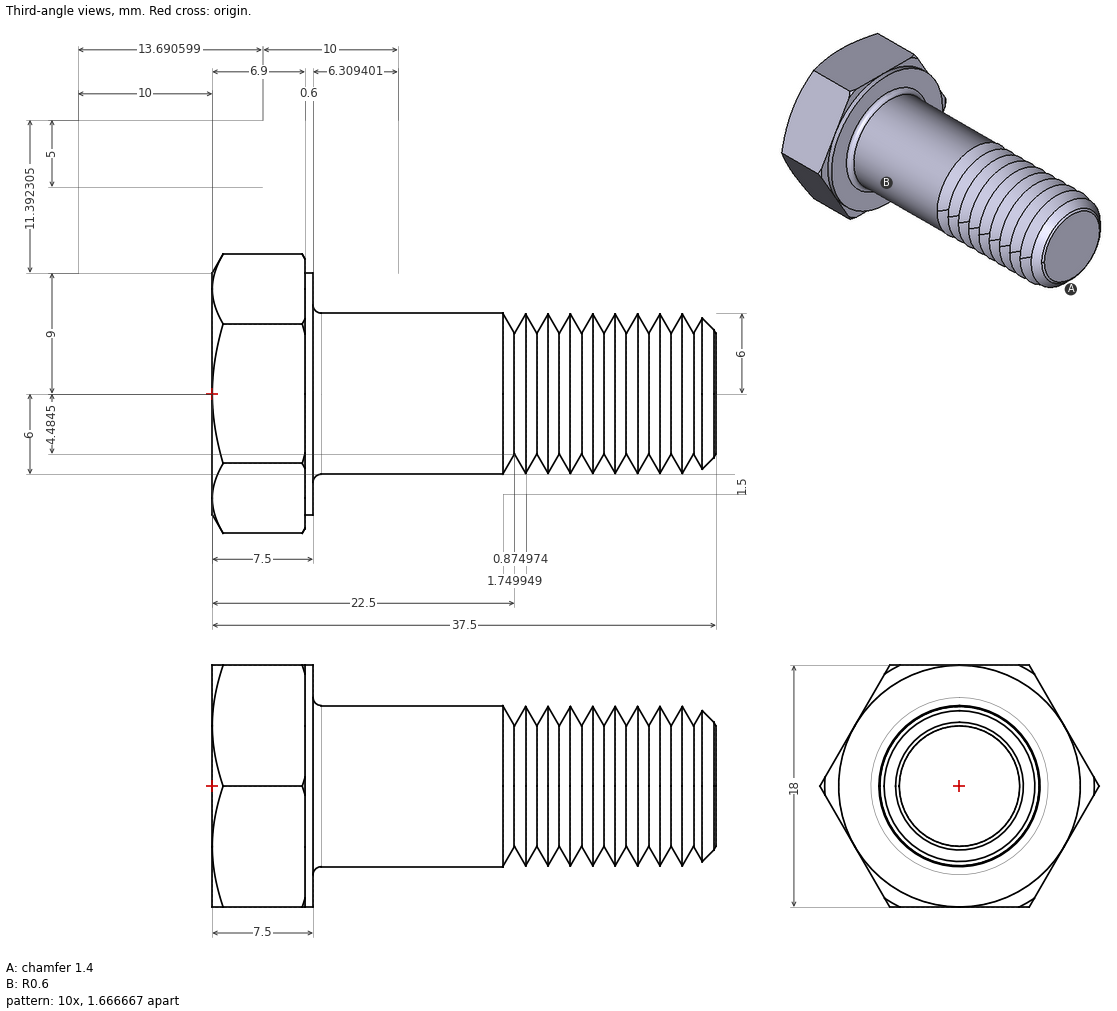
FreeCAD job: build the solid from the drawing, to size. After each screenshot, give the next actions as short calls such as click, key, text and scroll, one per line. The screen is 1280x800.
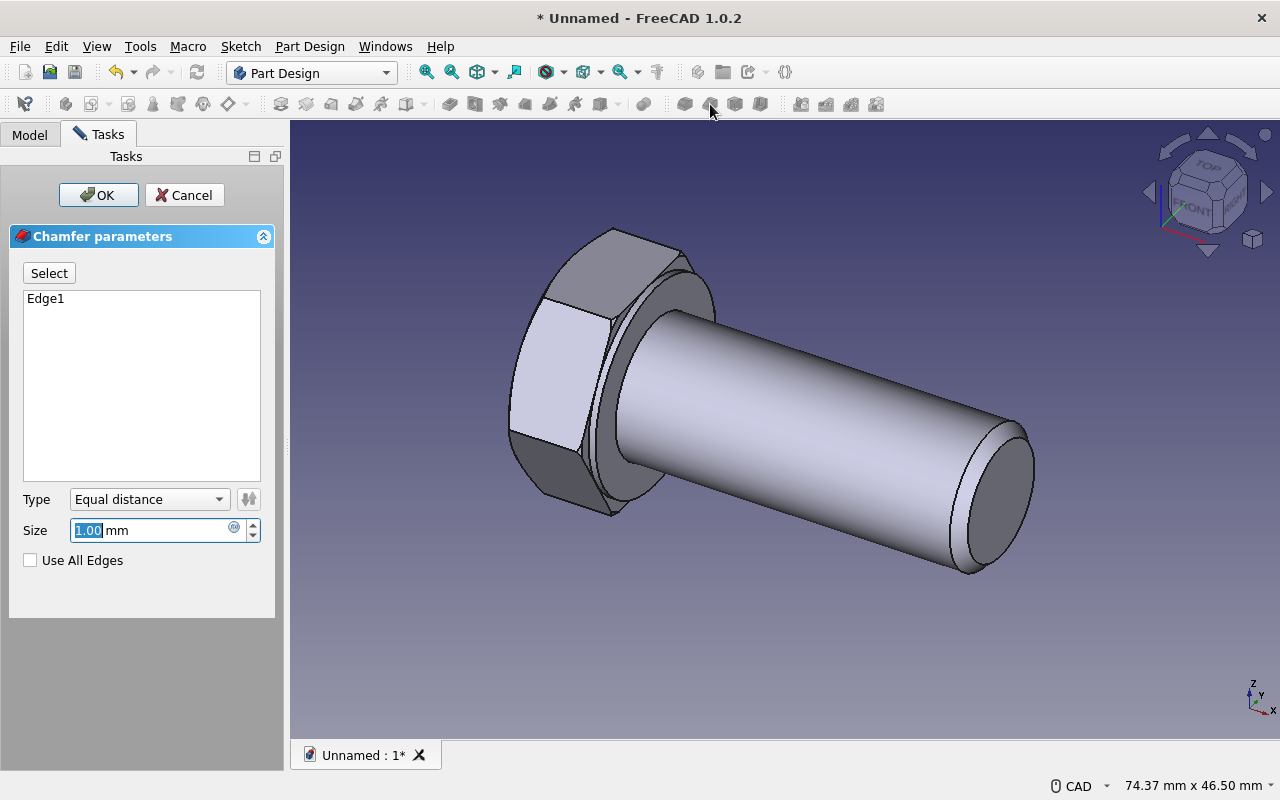
text(1.4)
key(Tab)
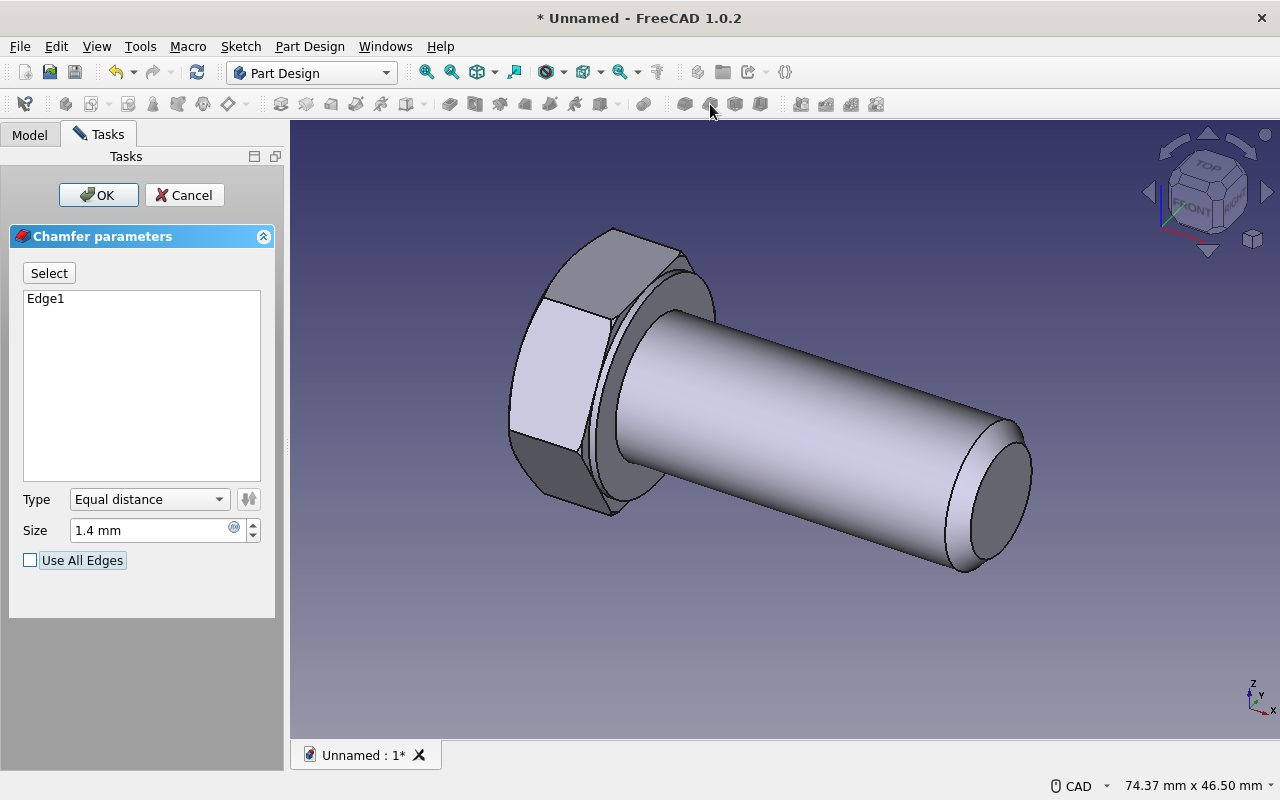
click(99, 195)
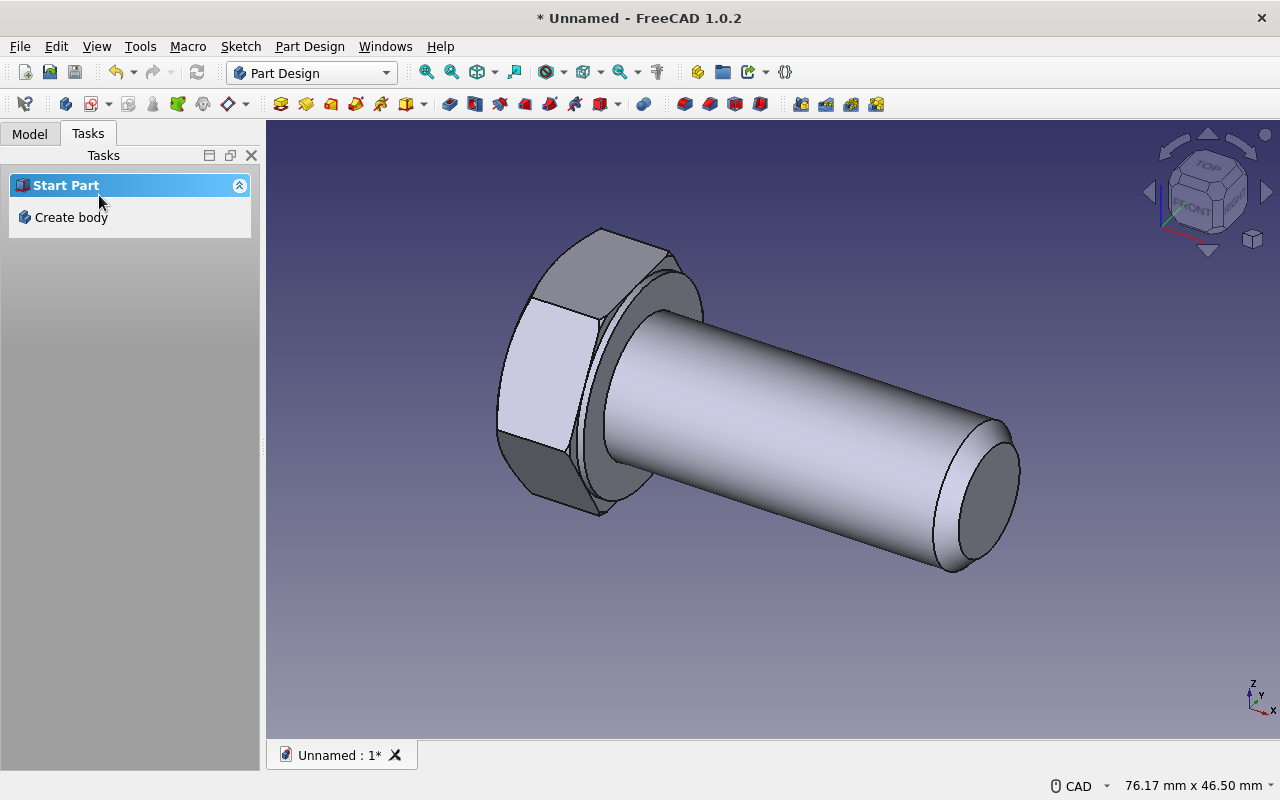
key(0)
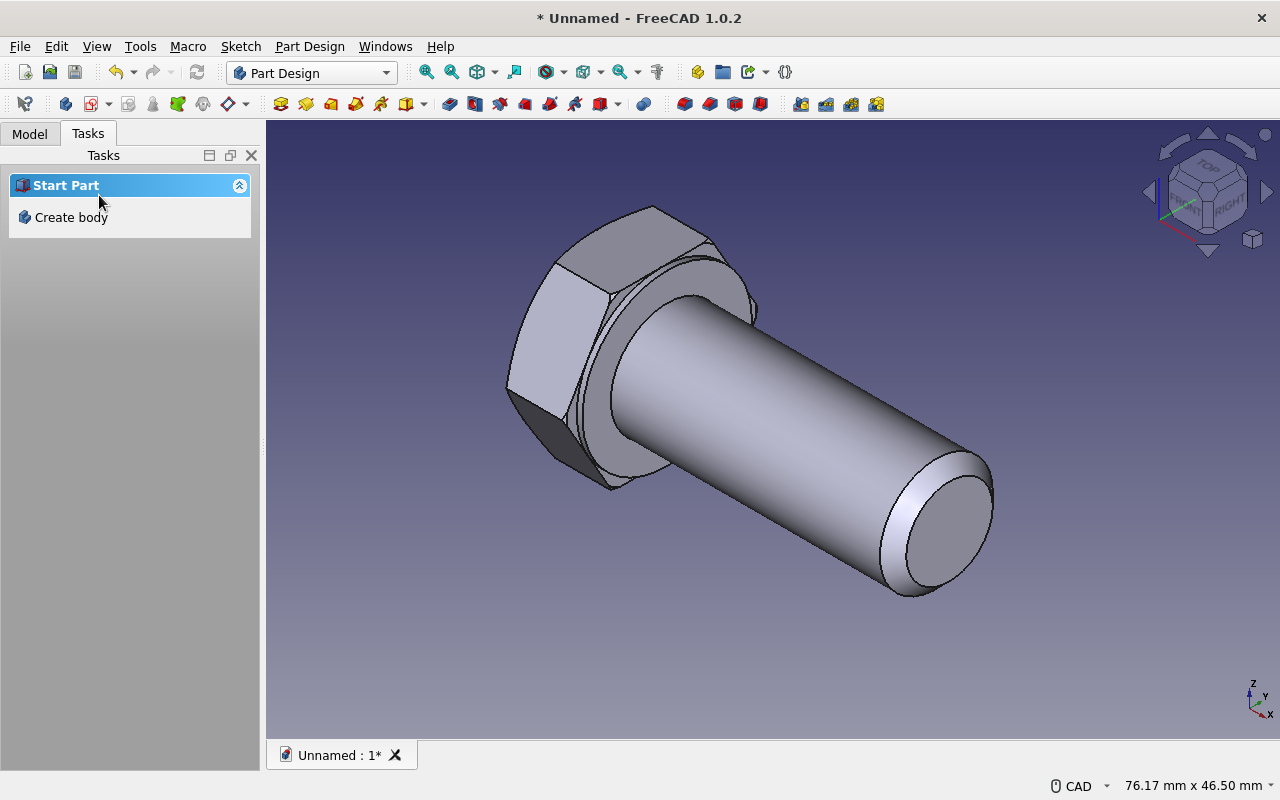
key(2)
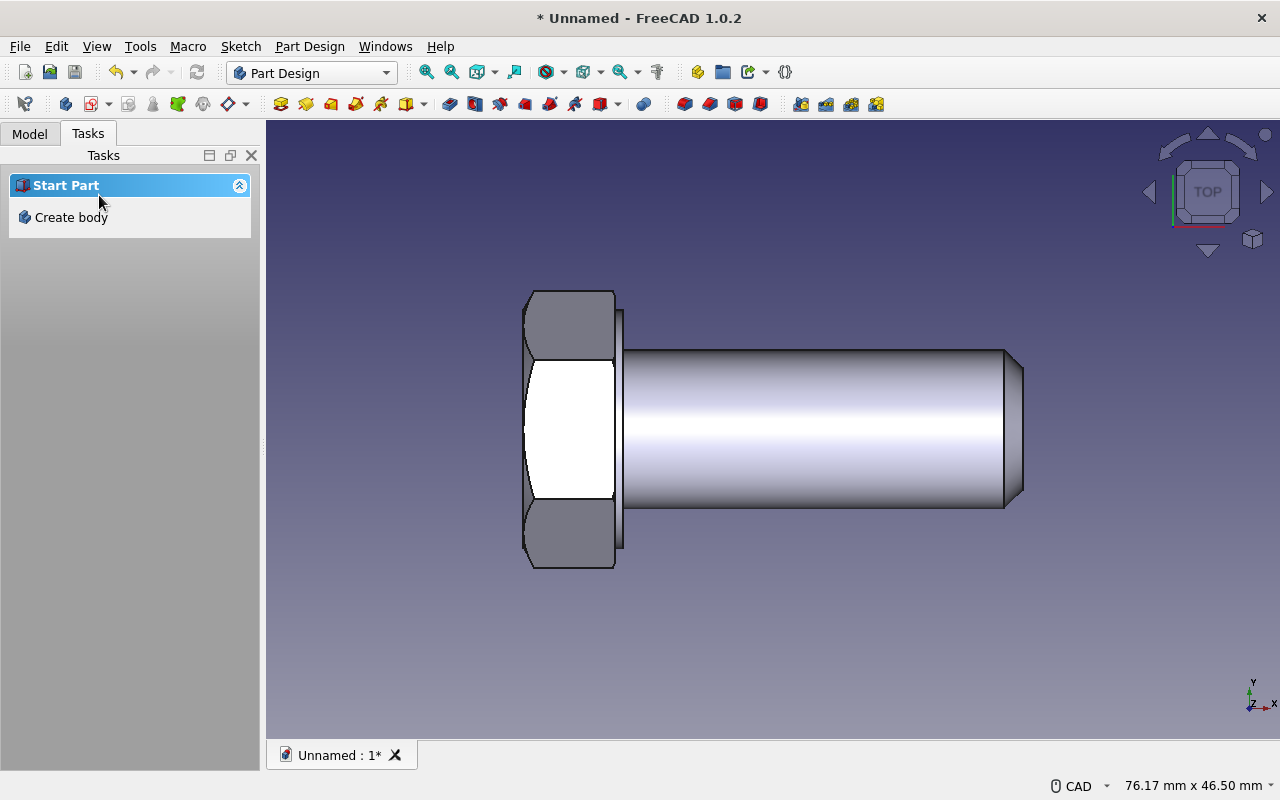
key(1)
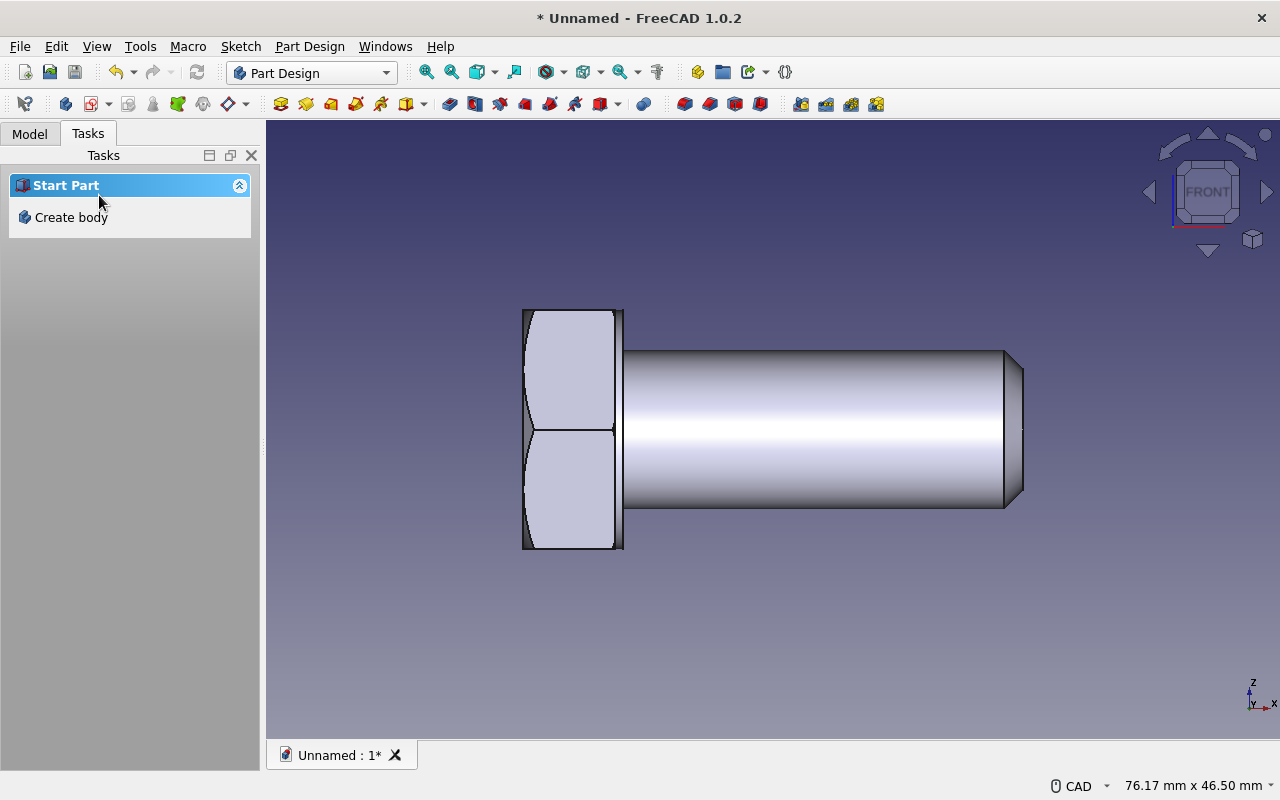
key(3)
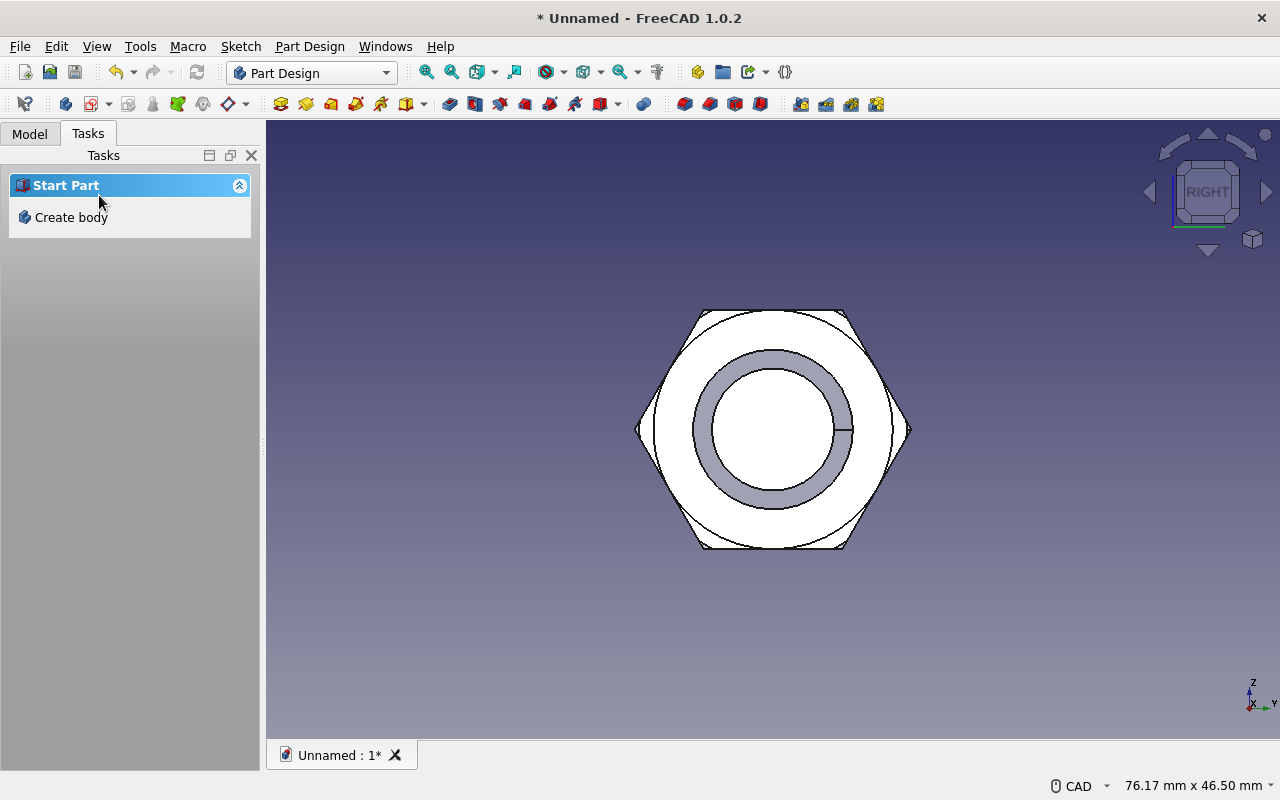
click(427, 72)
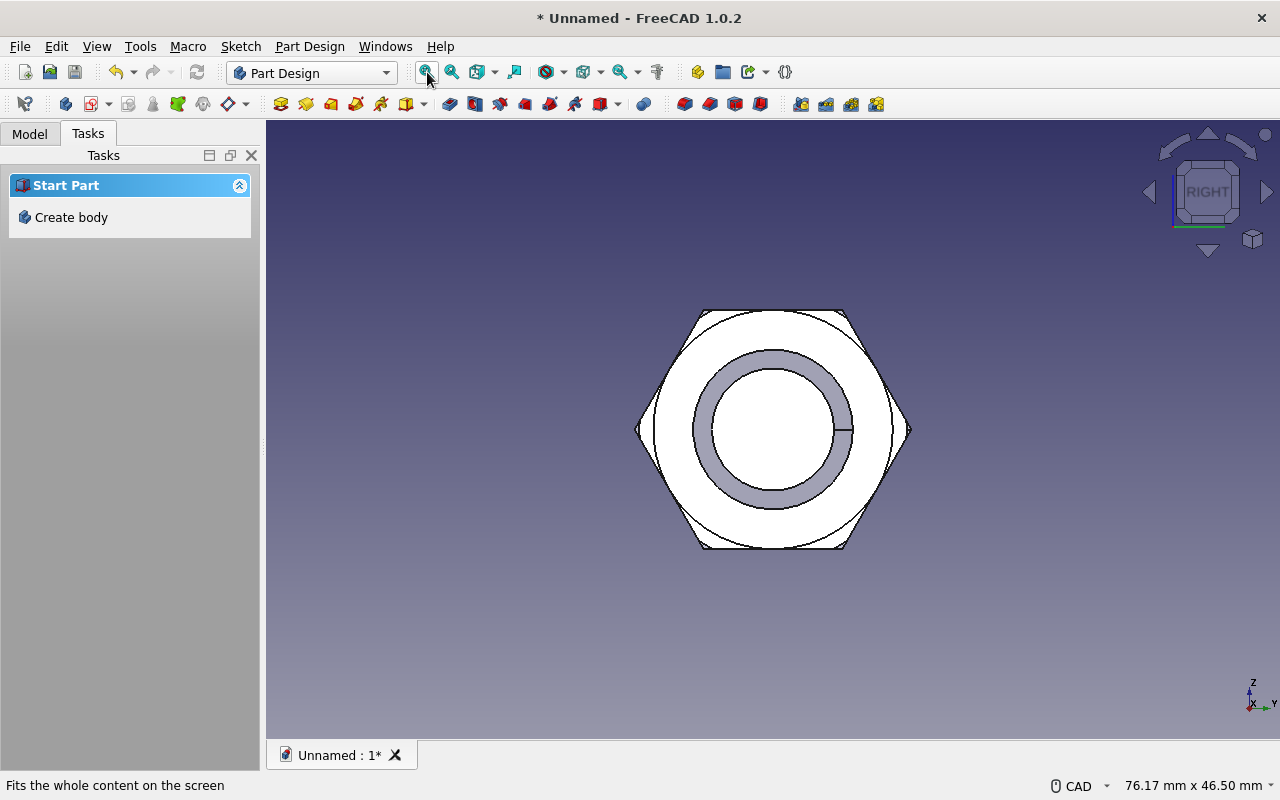
key(5)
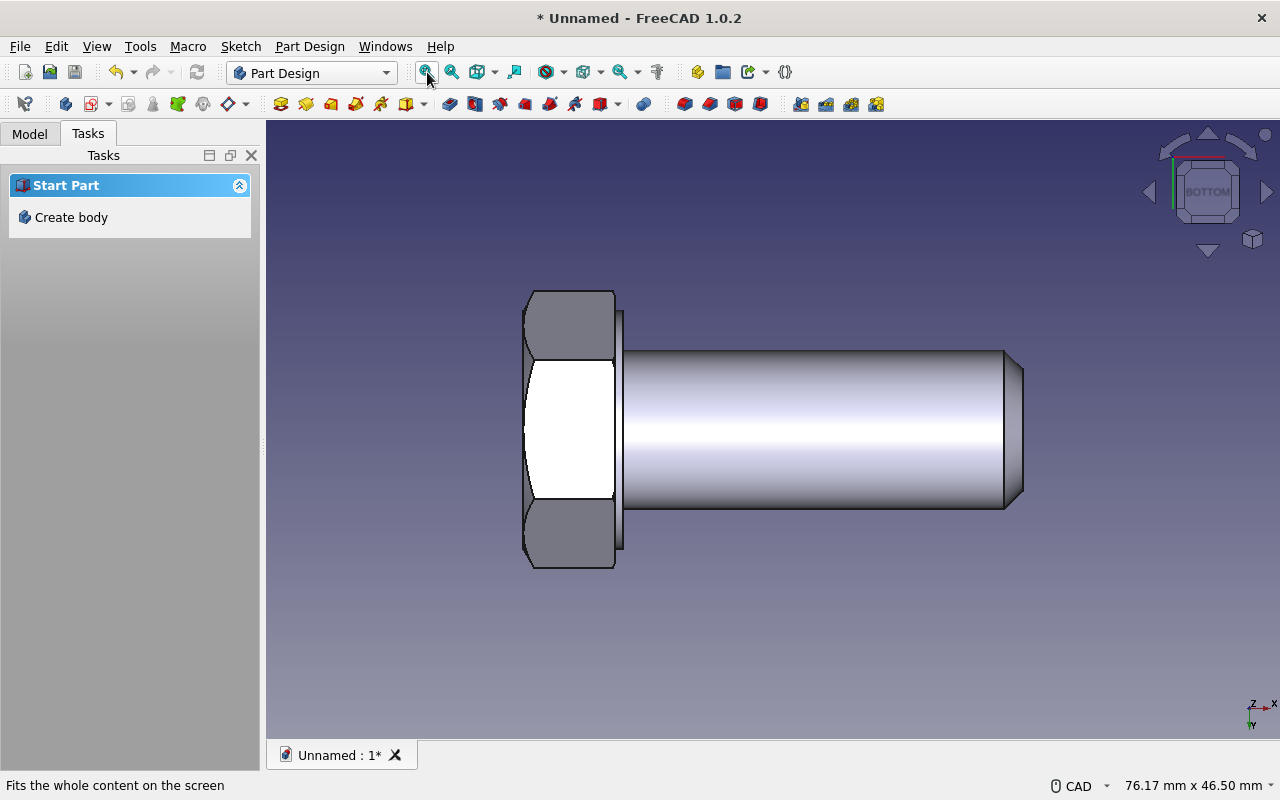
key(4)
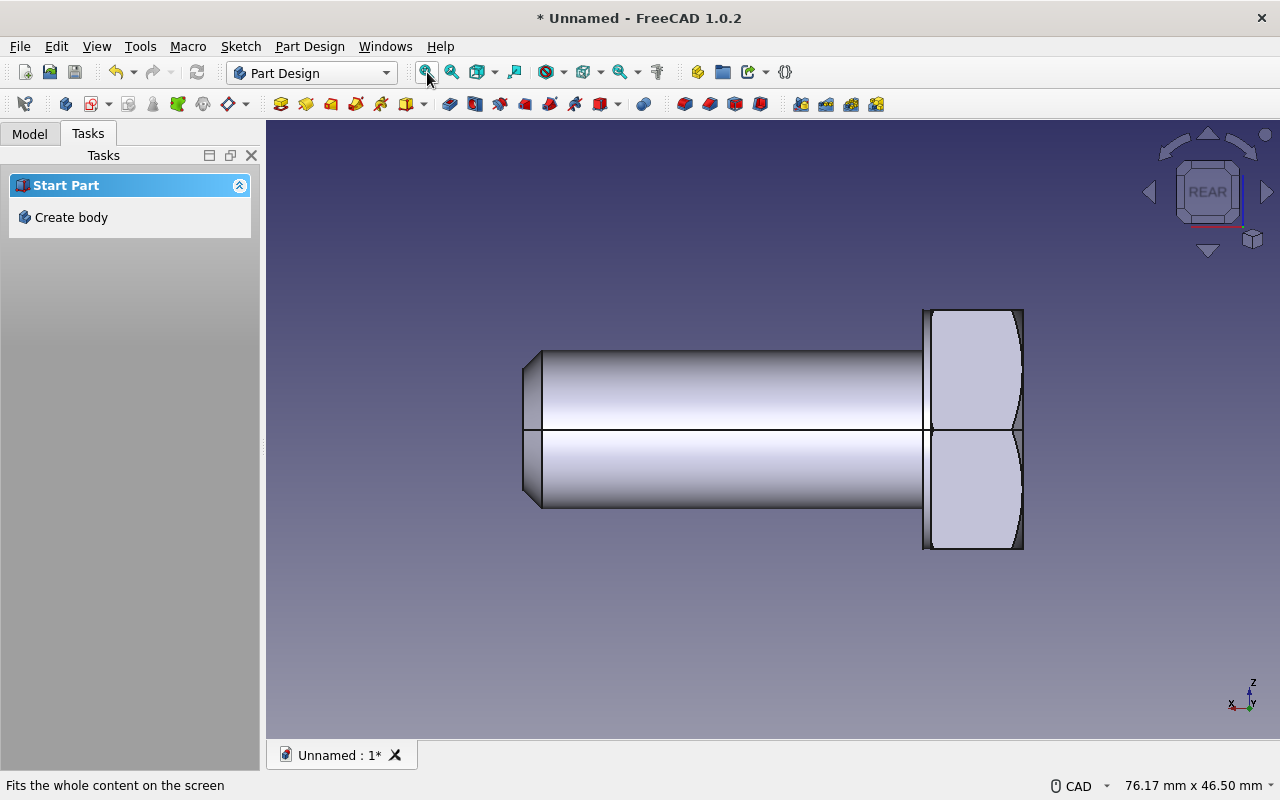
key(6)